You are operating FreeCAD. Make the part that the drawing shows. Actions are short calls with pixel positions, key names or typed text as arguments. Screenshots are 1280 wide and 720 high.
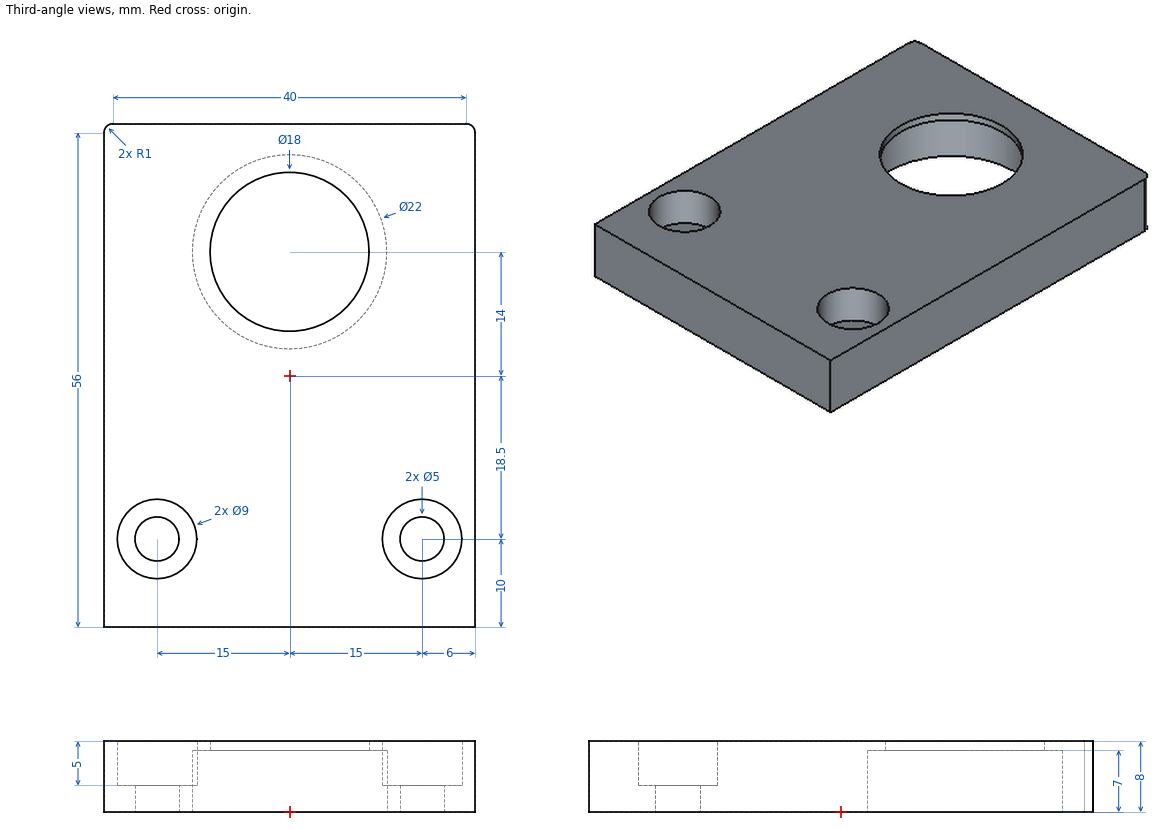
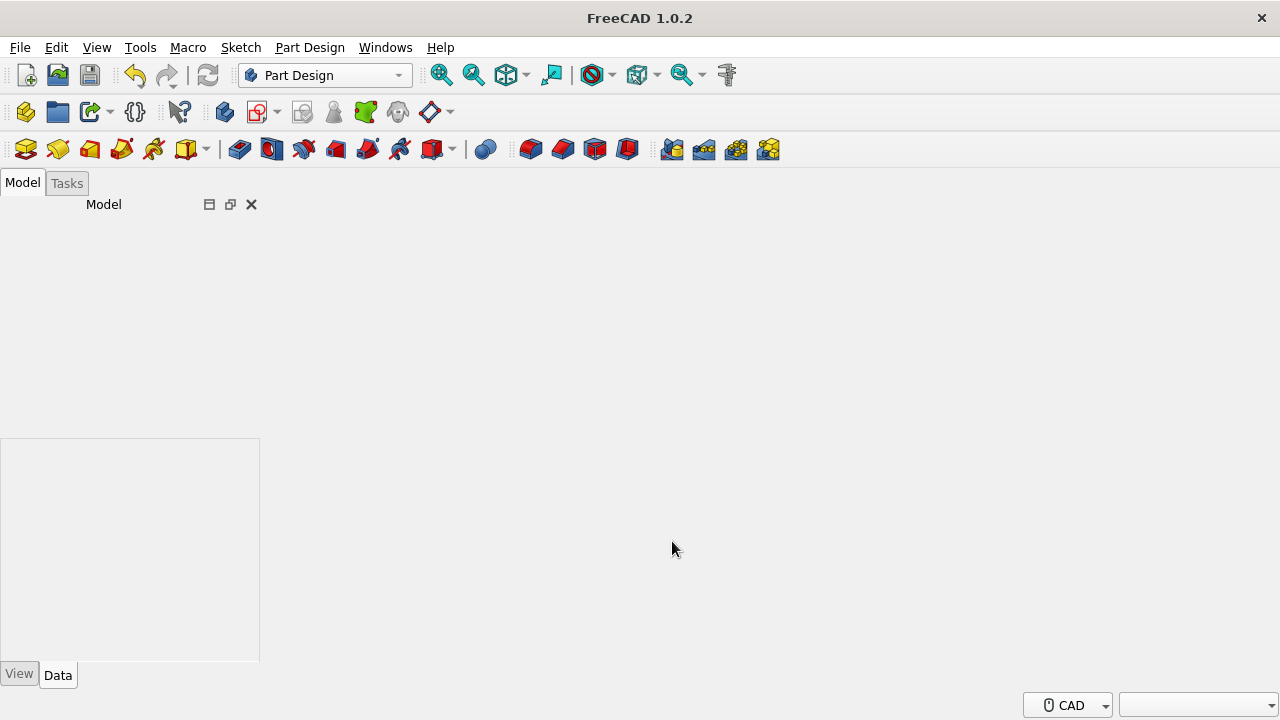
click(26, 76)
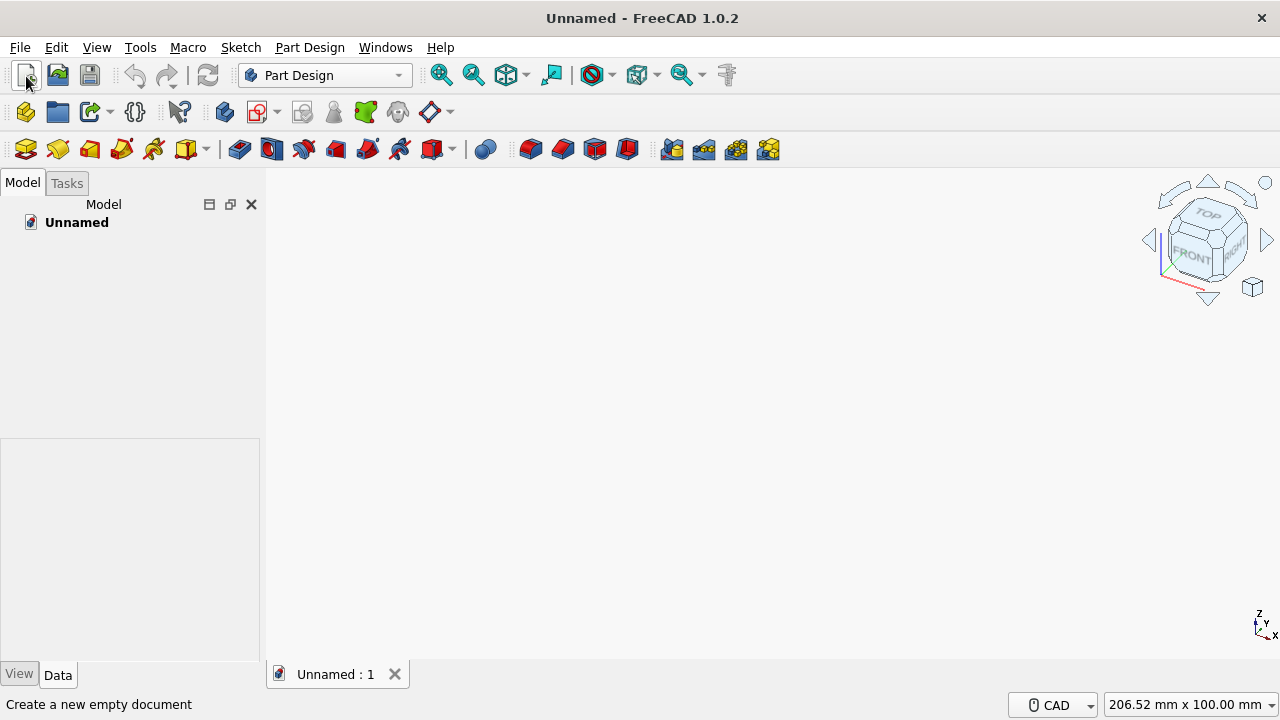
click(258, 112)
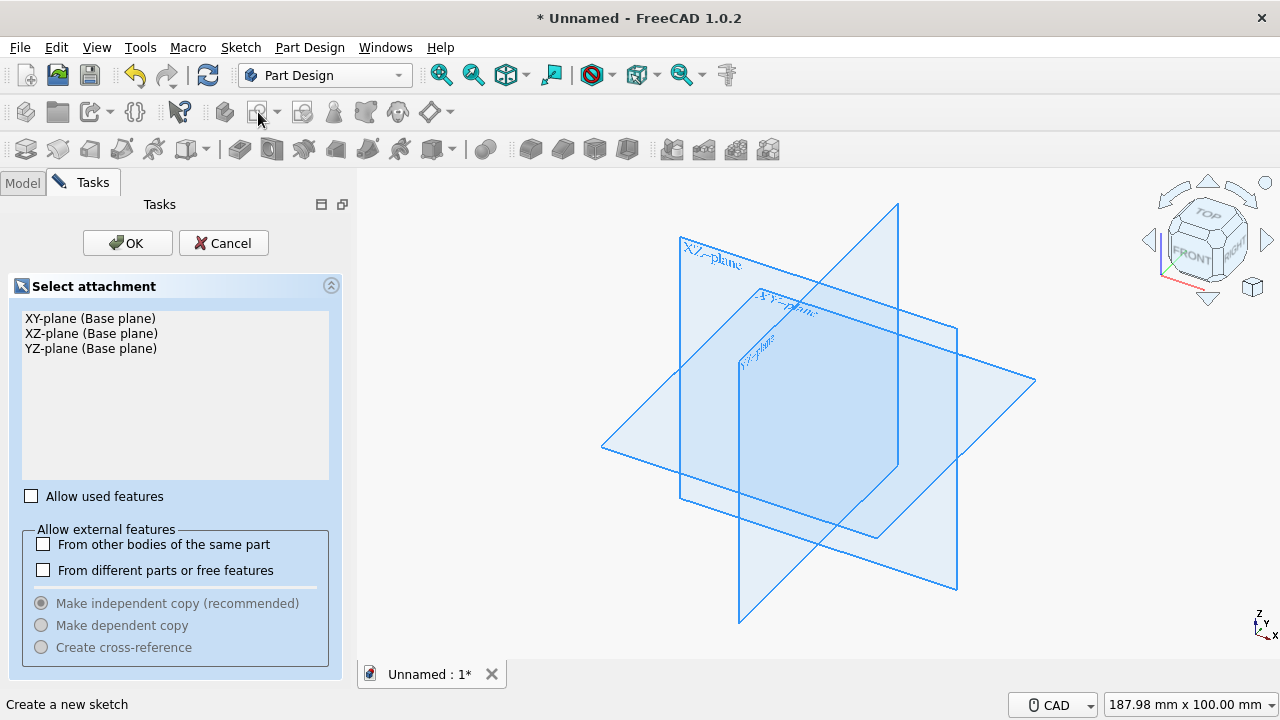
click(82, 318)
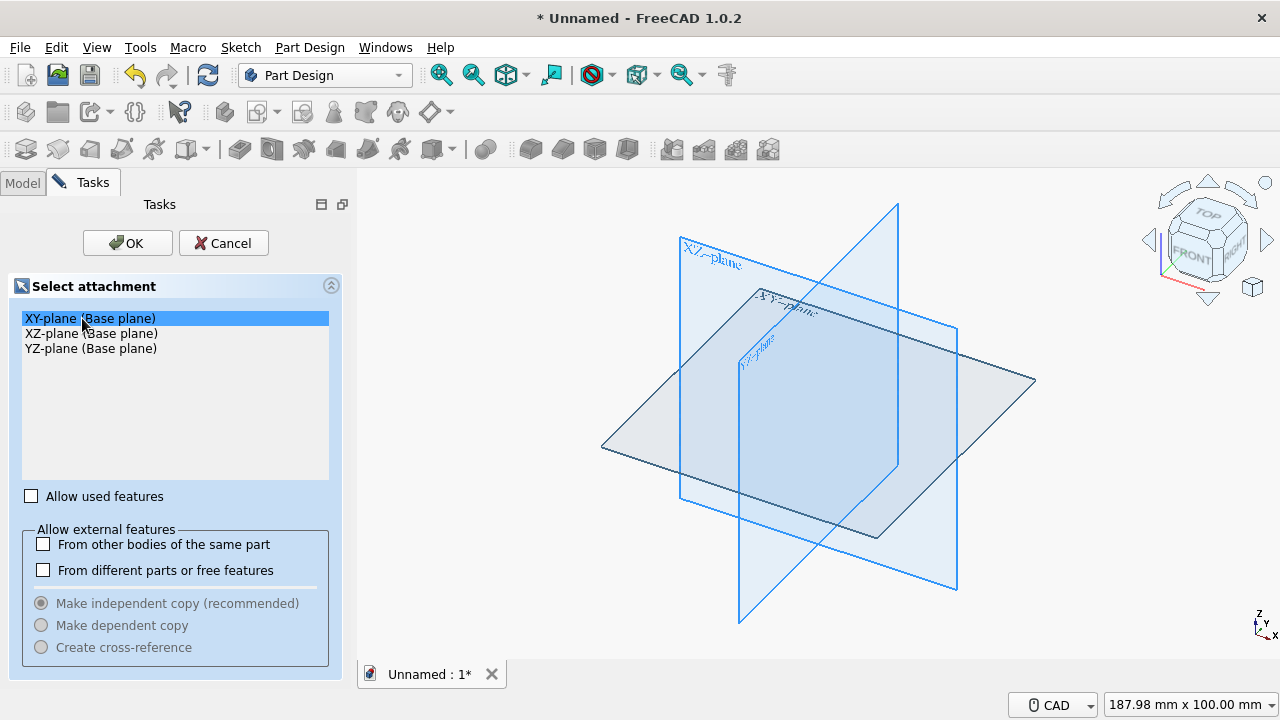
click(128, 243)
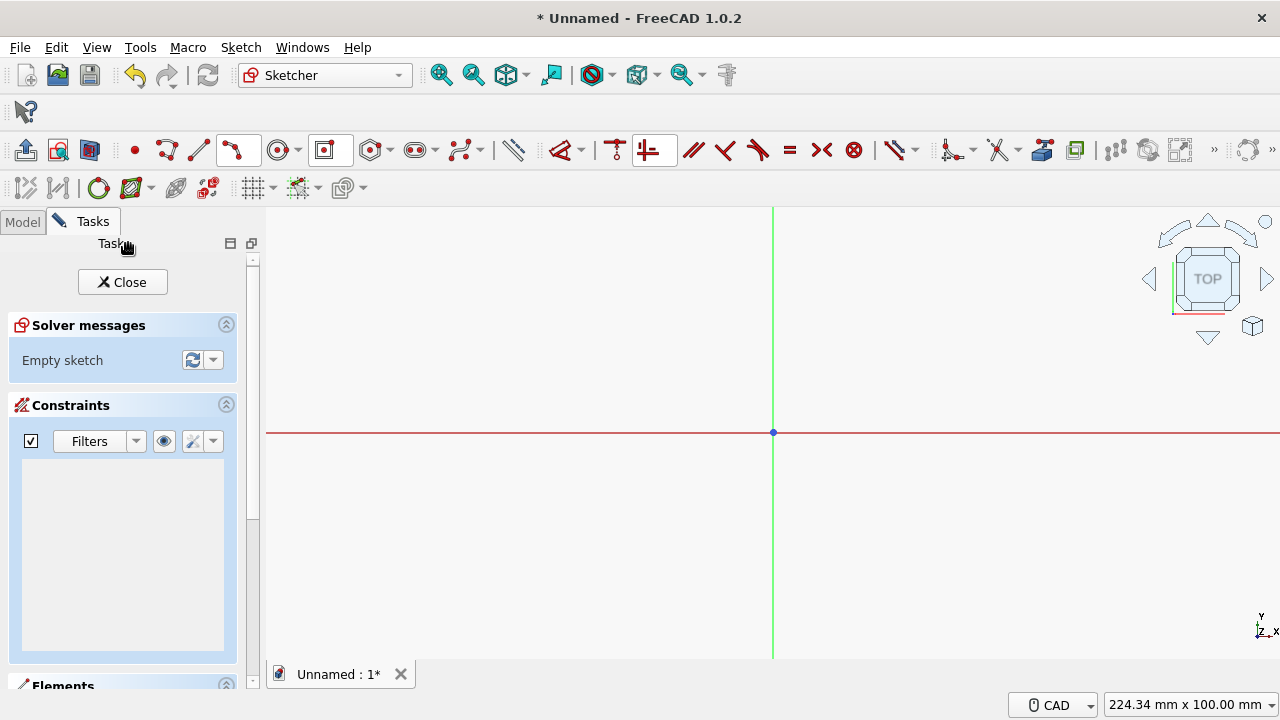
click(200, 150)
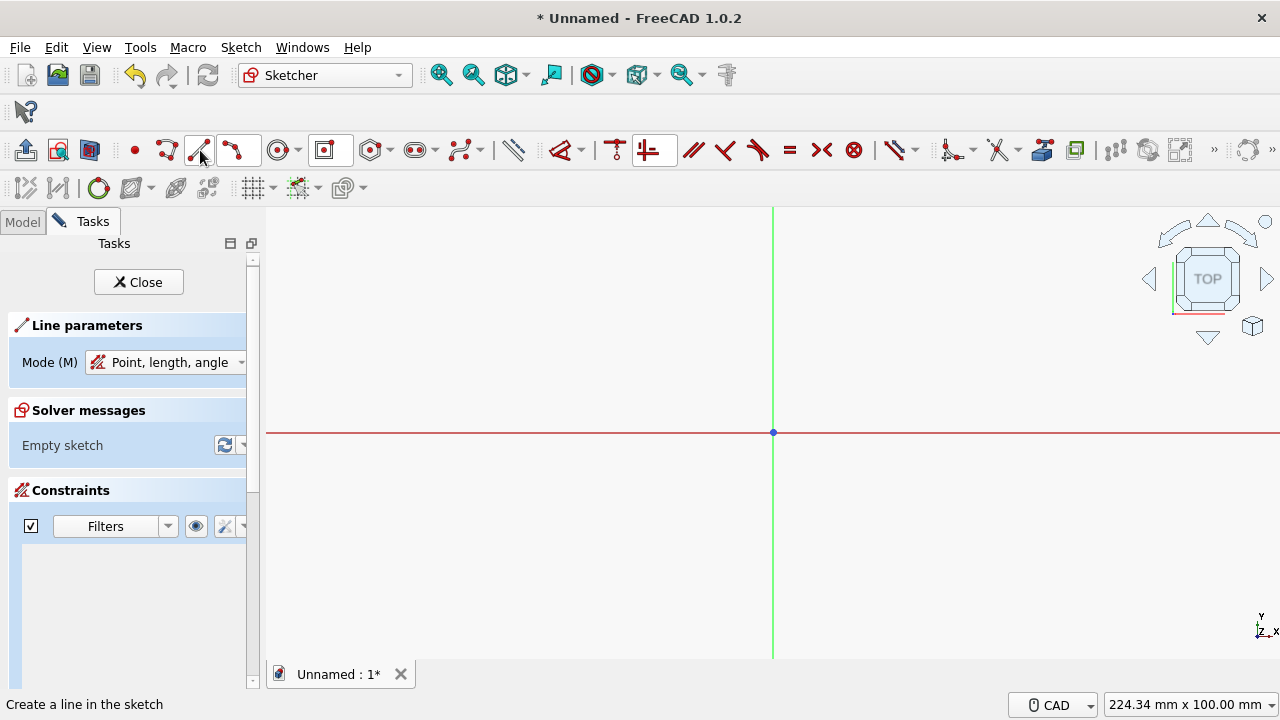
click(863, 304)
click(683, 304)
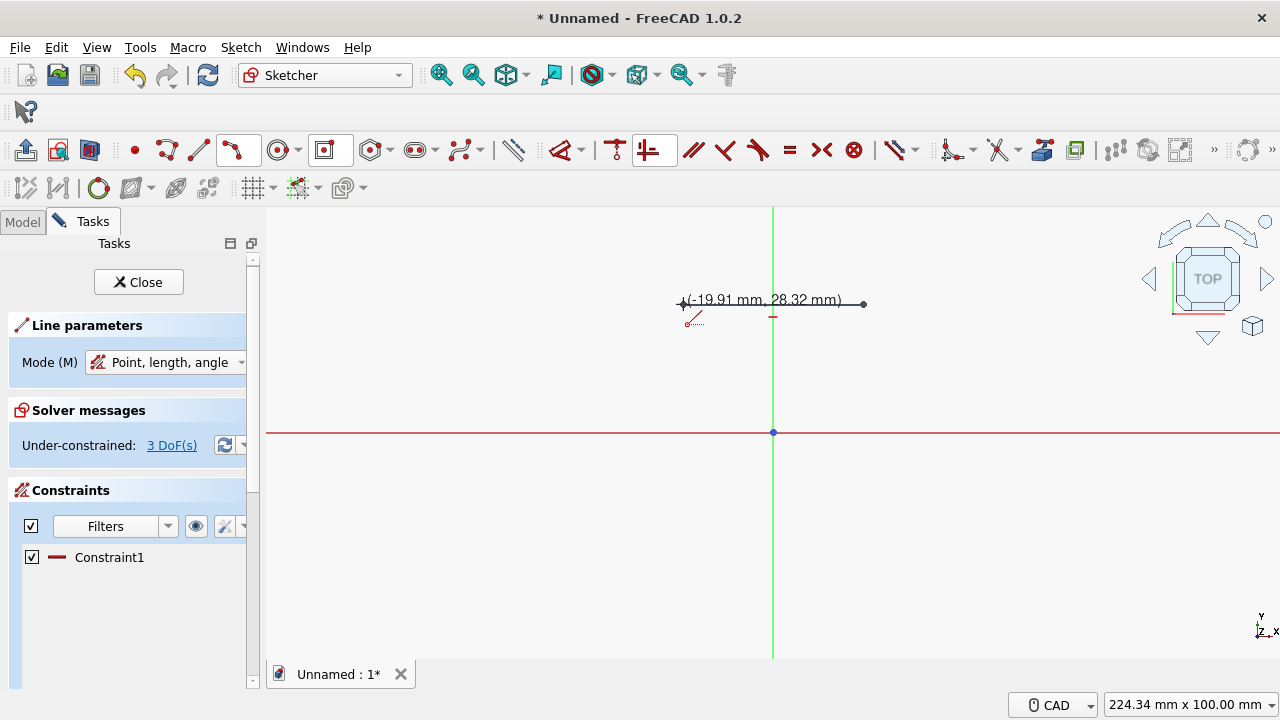
click(168, 150)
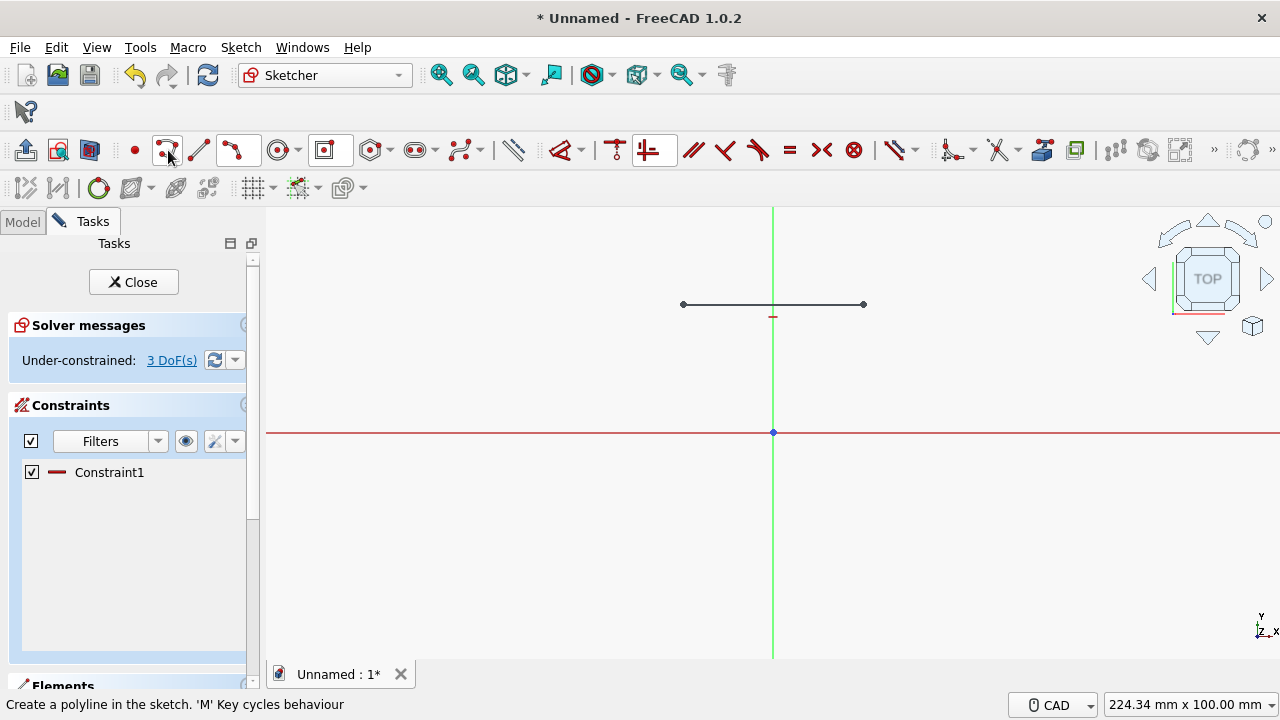
scroll(678, 309, up, 5)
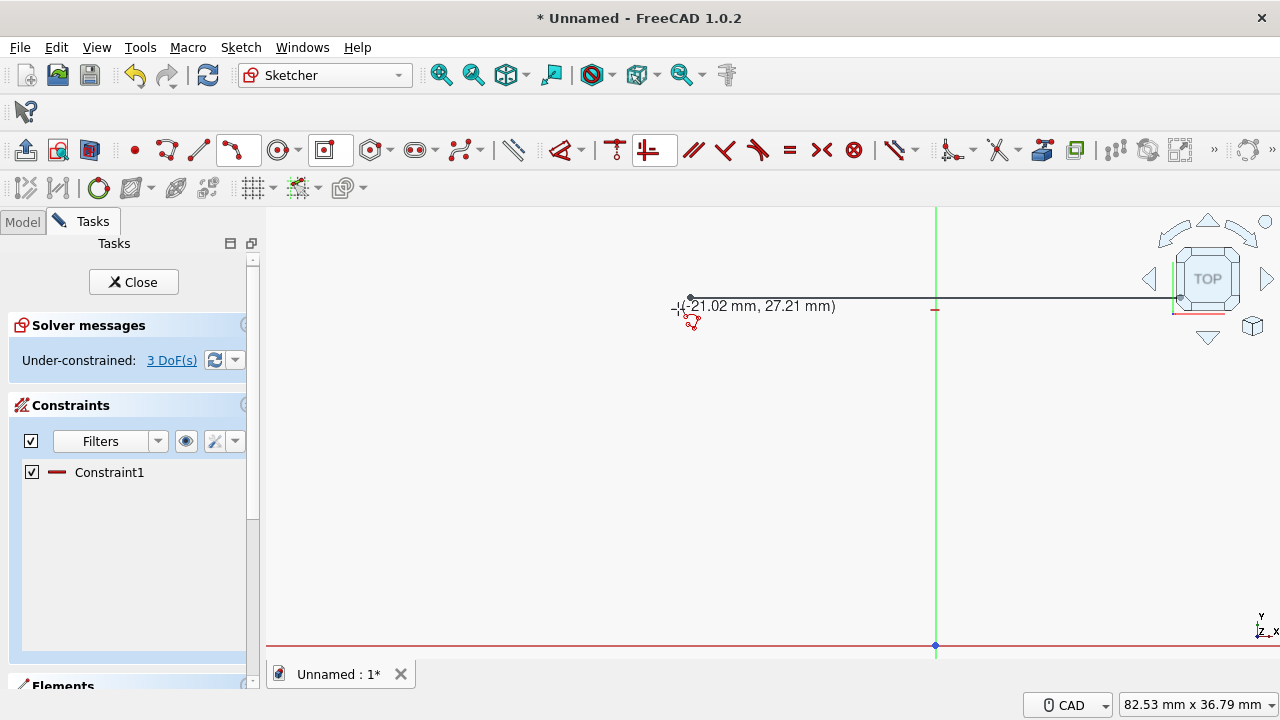
click(678, 308)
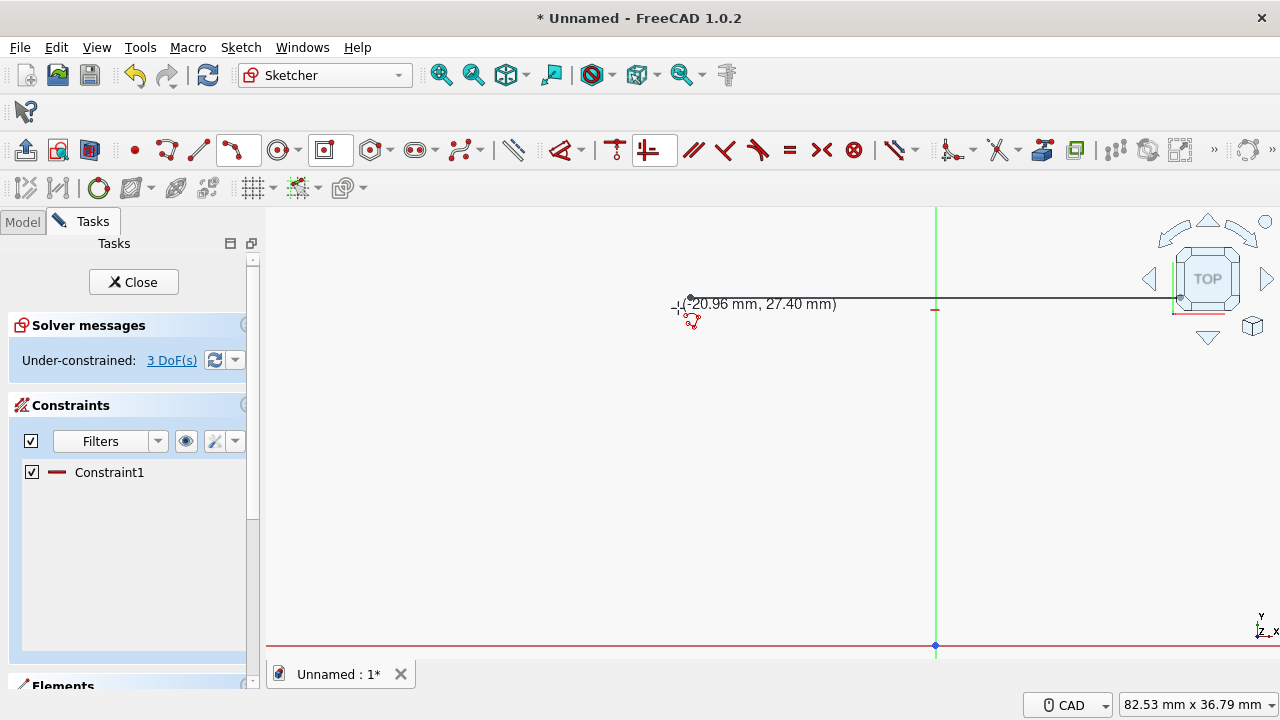
scroll(570, 309, down, 5)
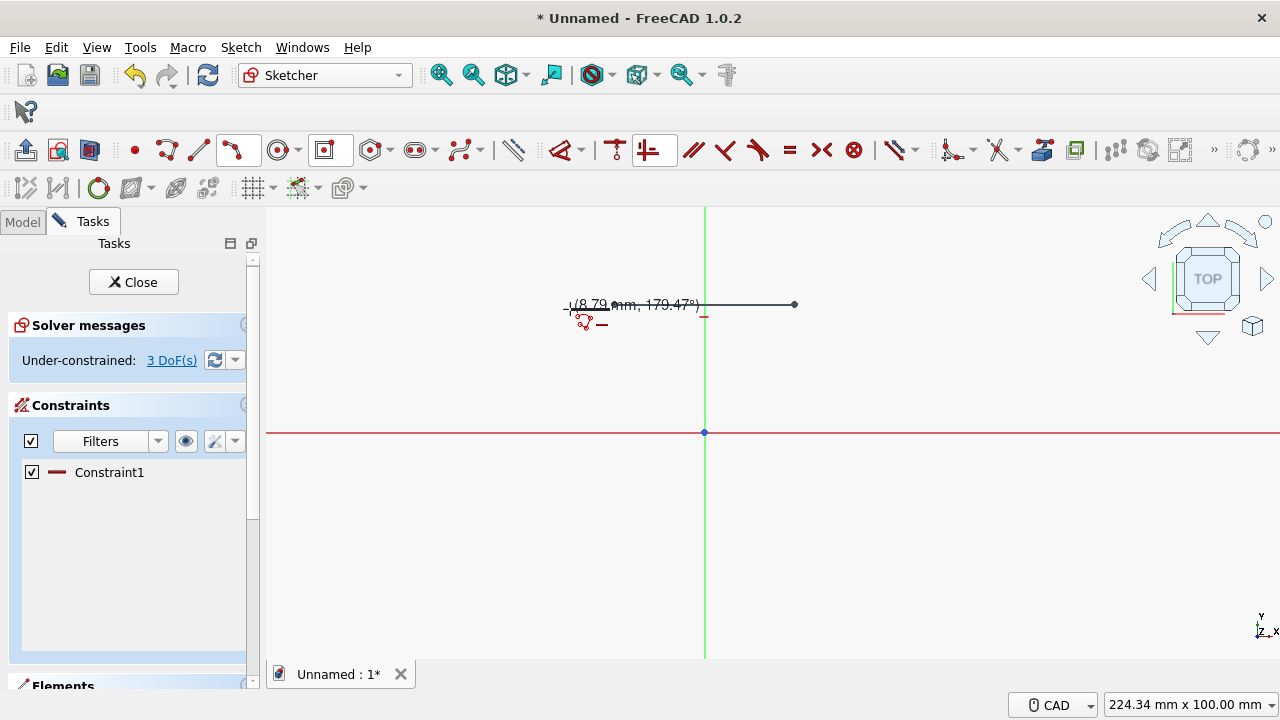
click(610, 562)
click(800, 562)